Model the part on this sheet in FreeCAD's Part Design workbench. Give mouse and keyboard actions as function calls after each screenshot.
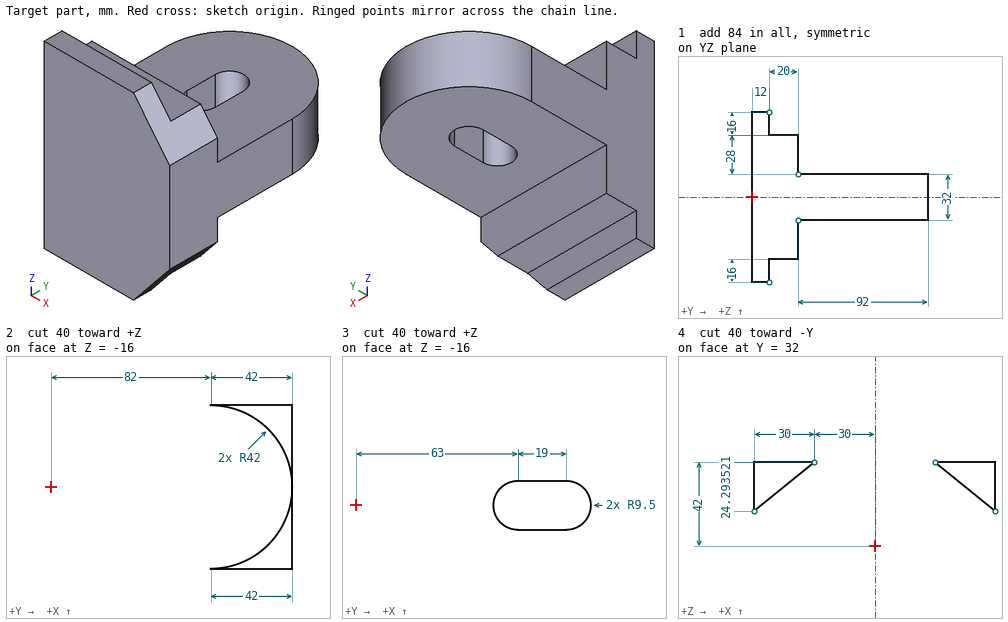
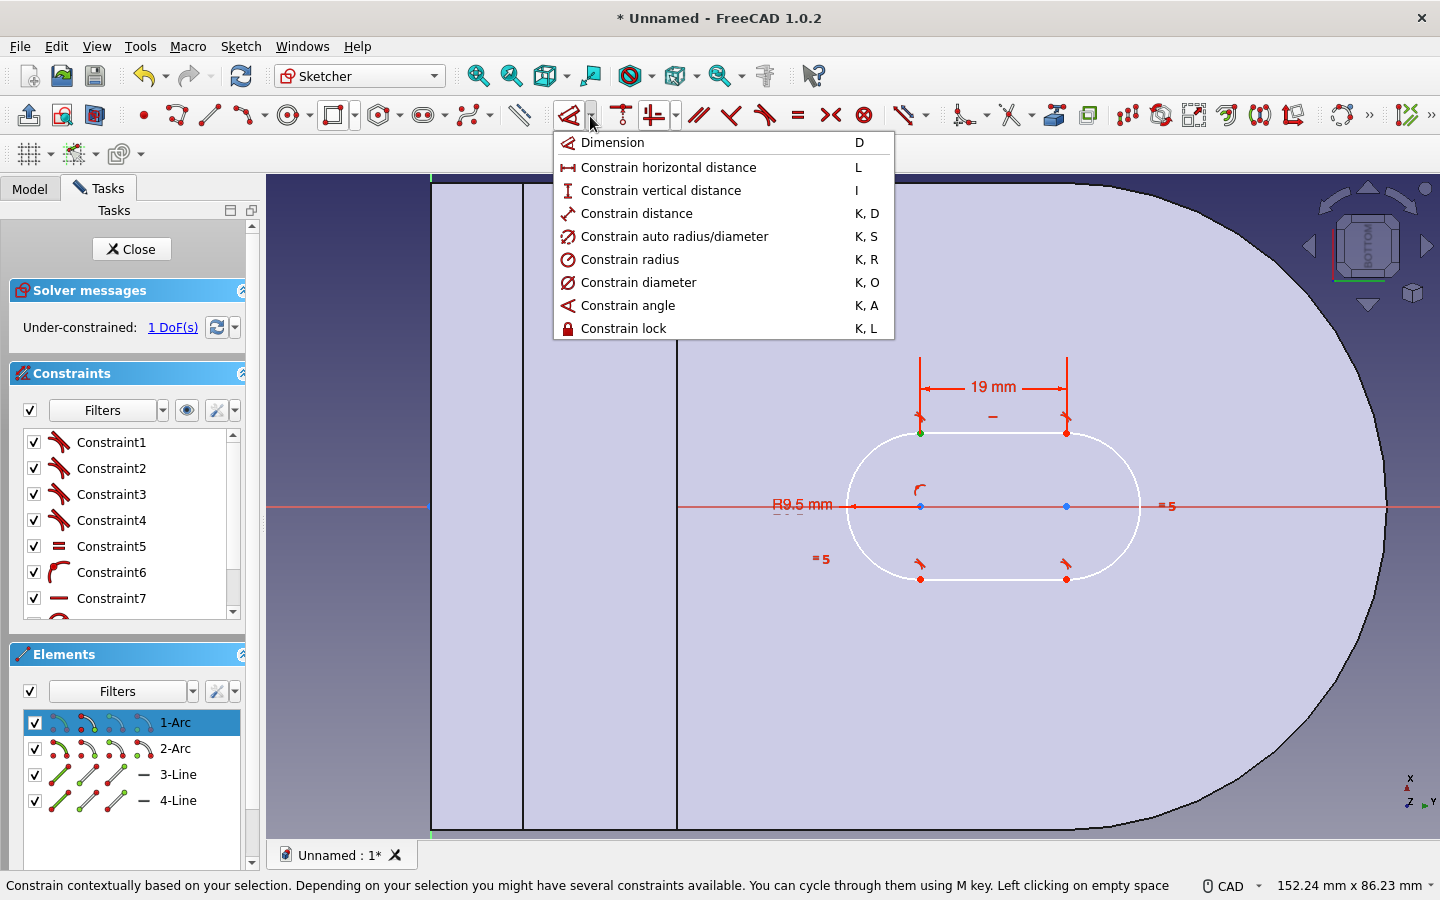
click(724, 168)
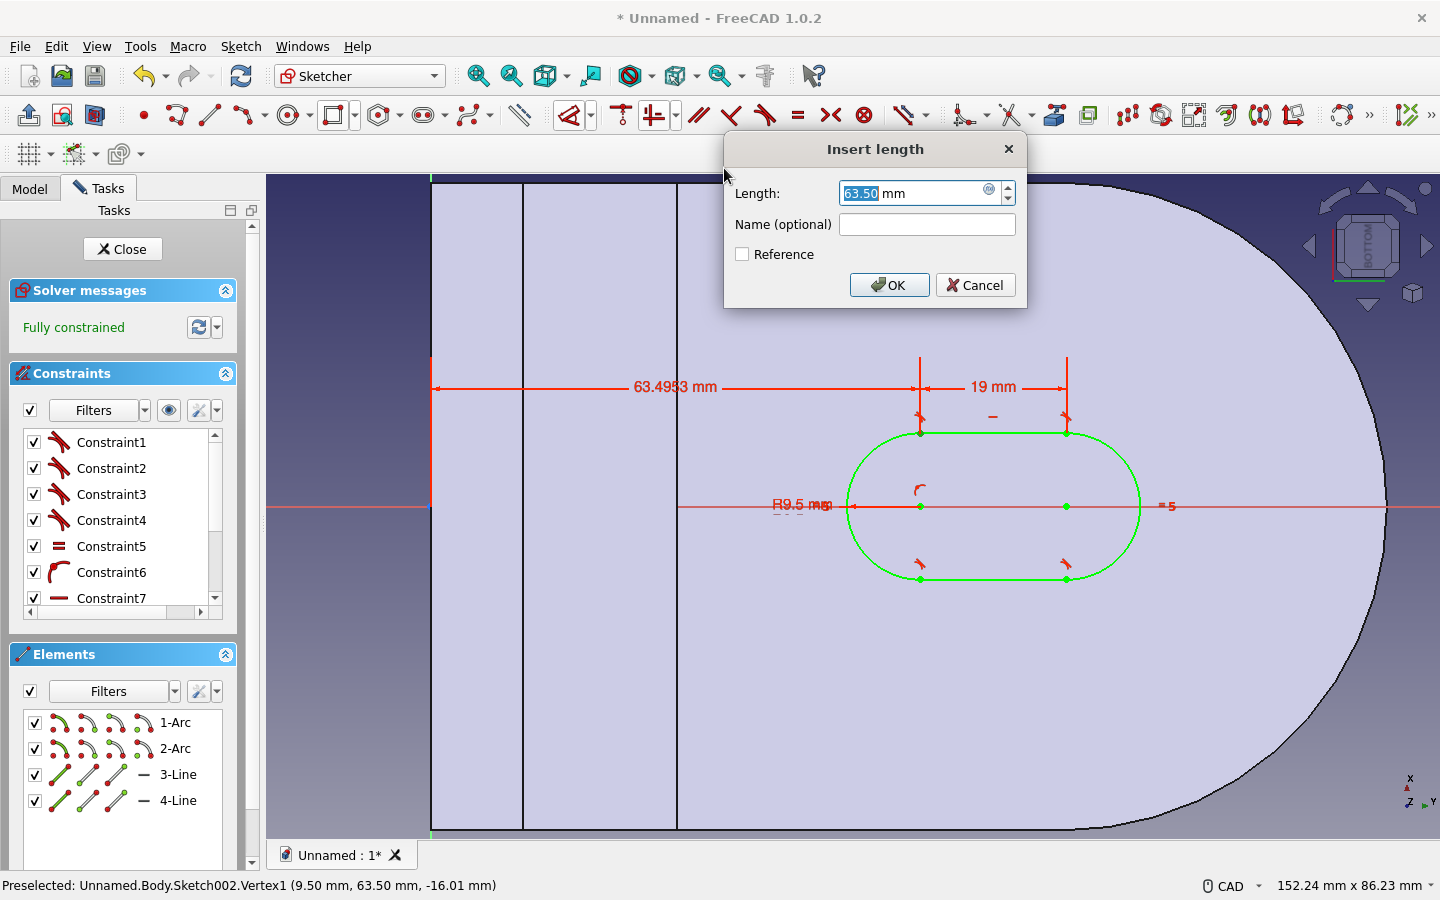
text(63)
key(Return)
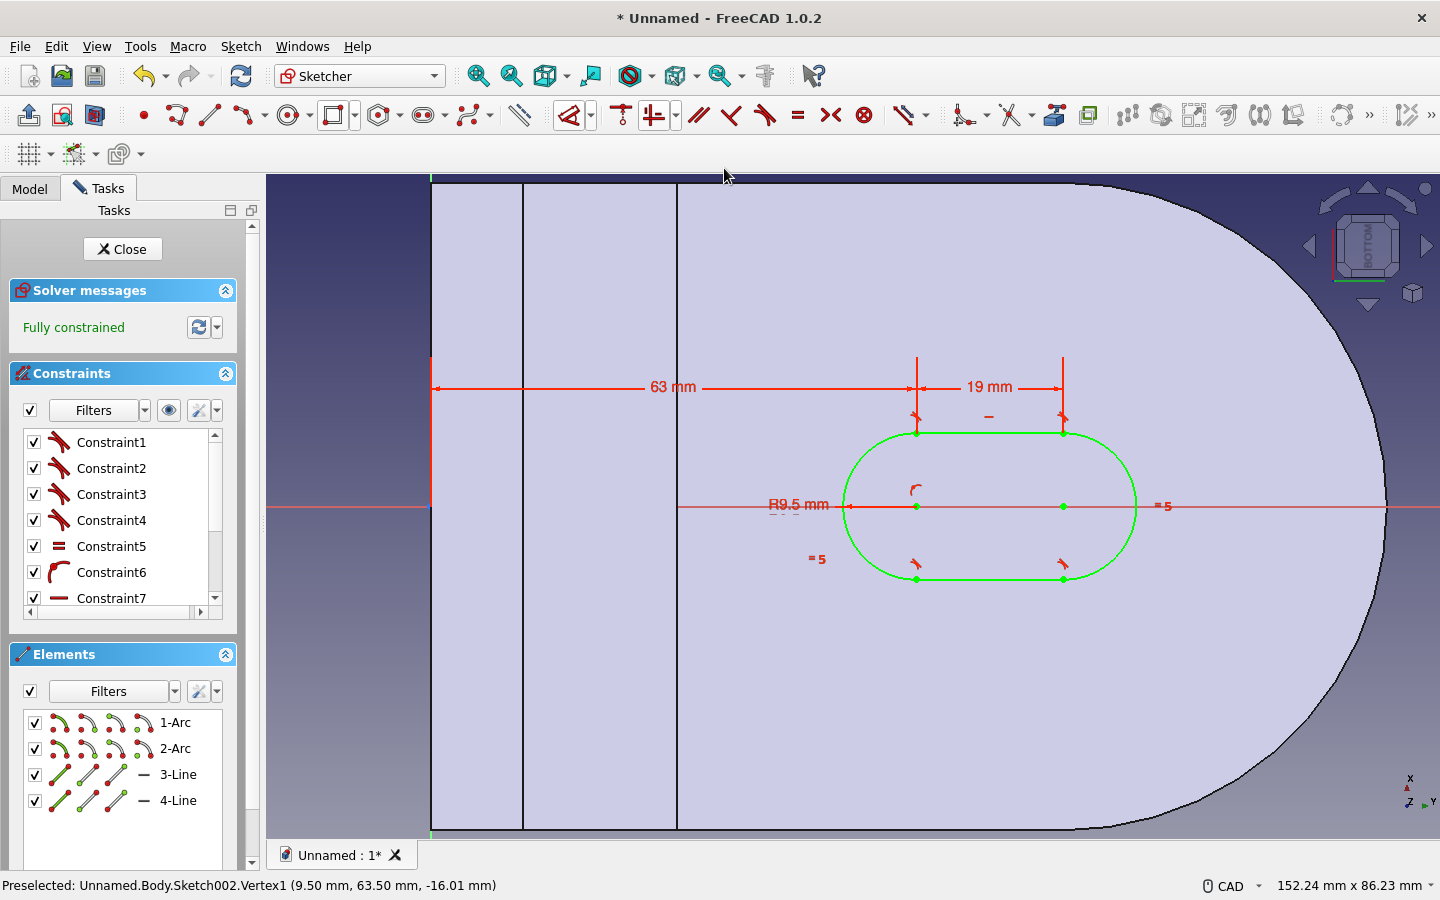
click(123, 249)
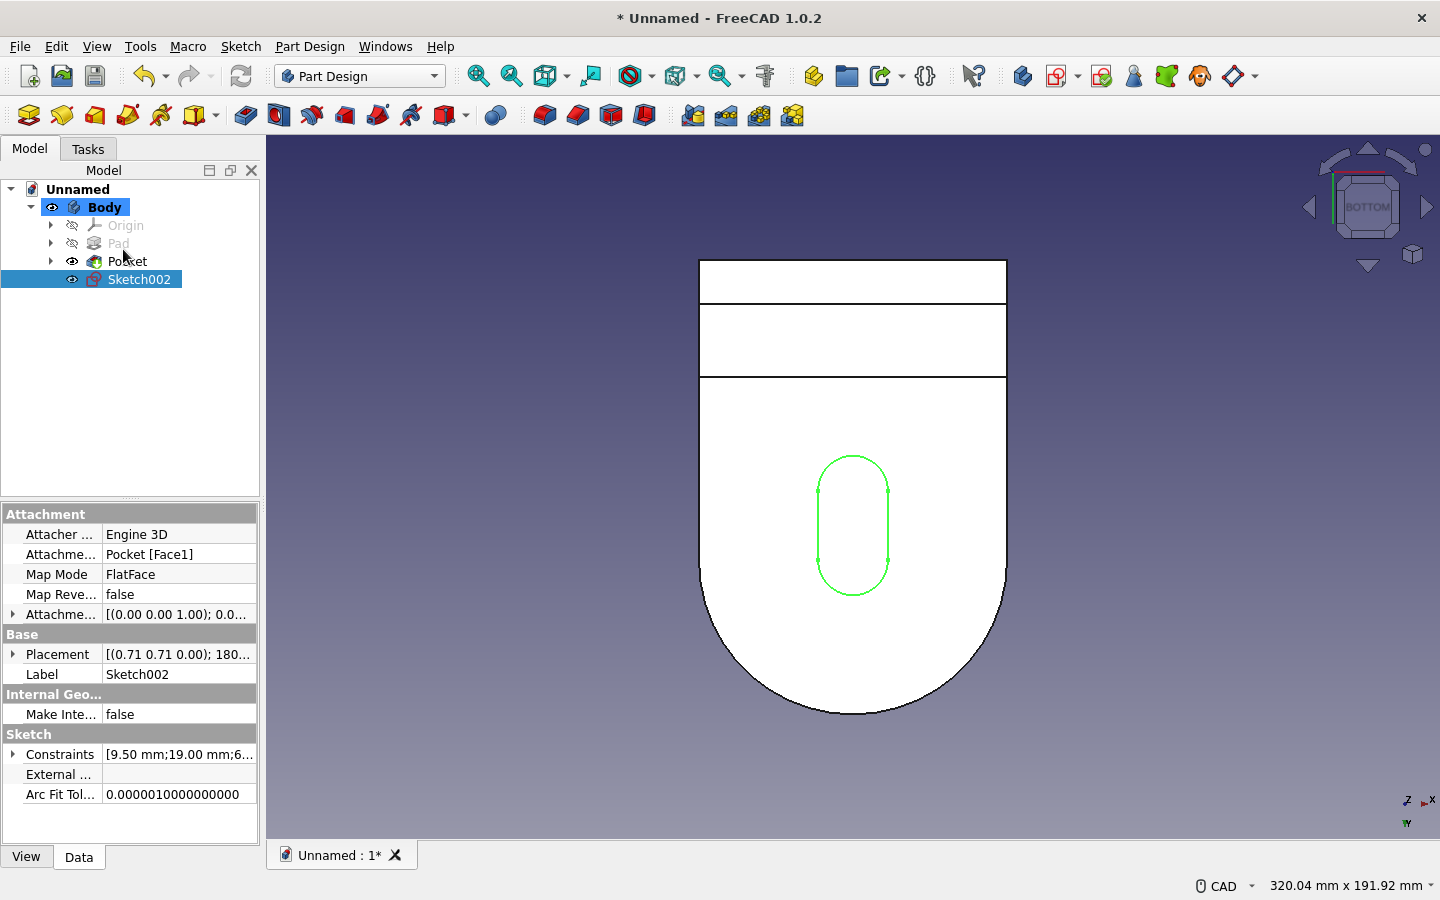
click(246, 116)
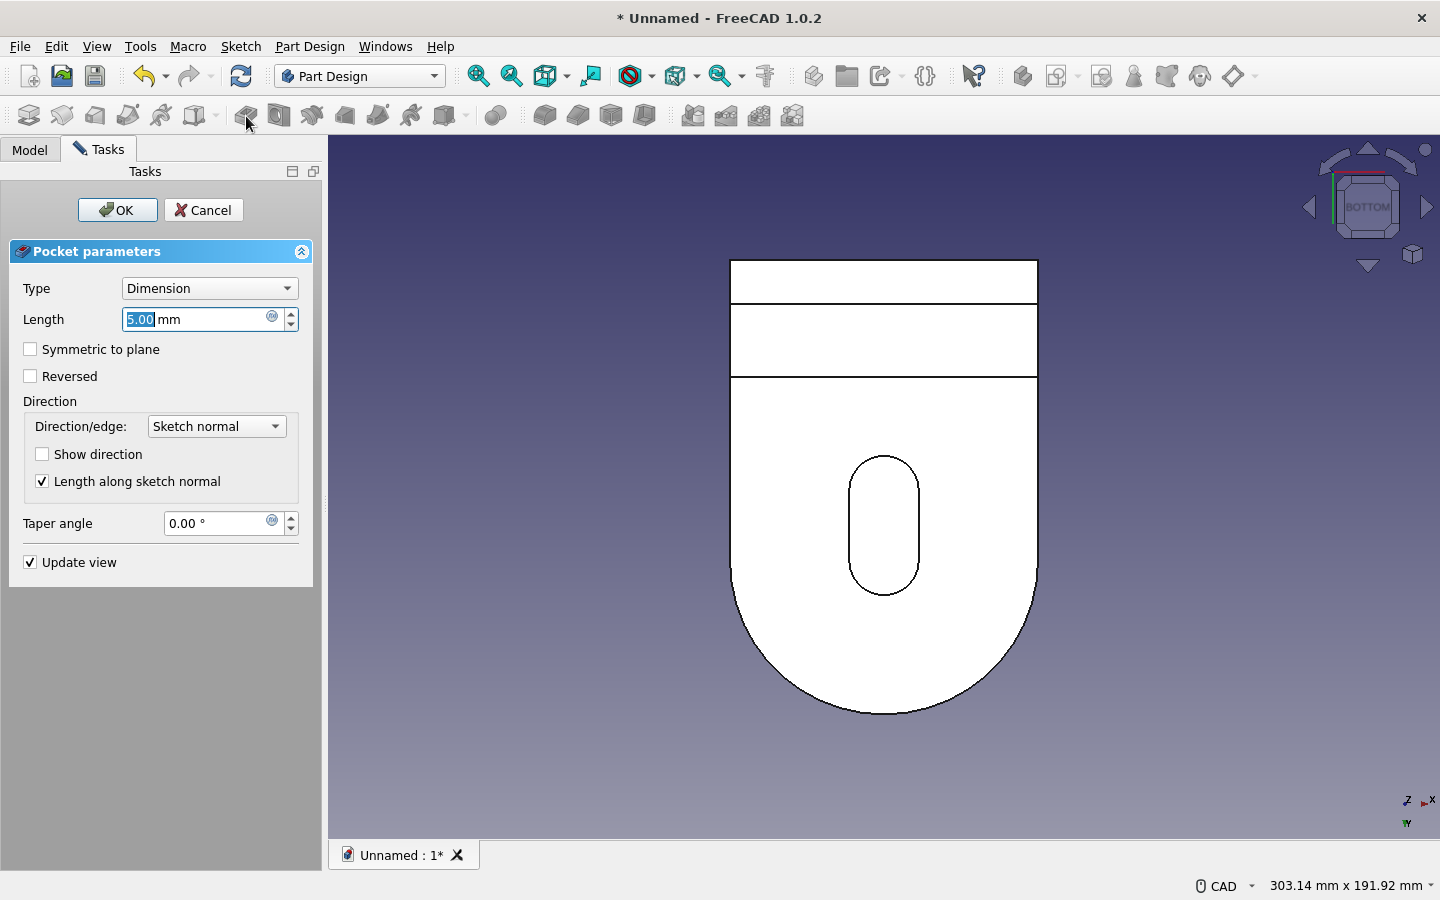
text(40)
key(Tab)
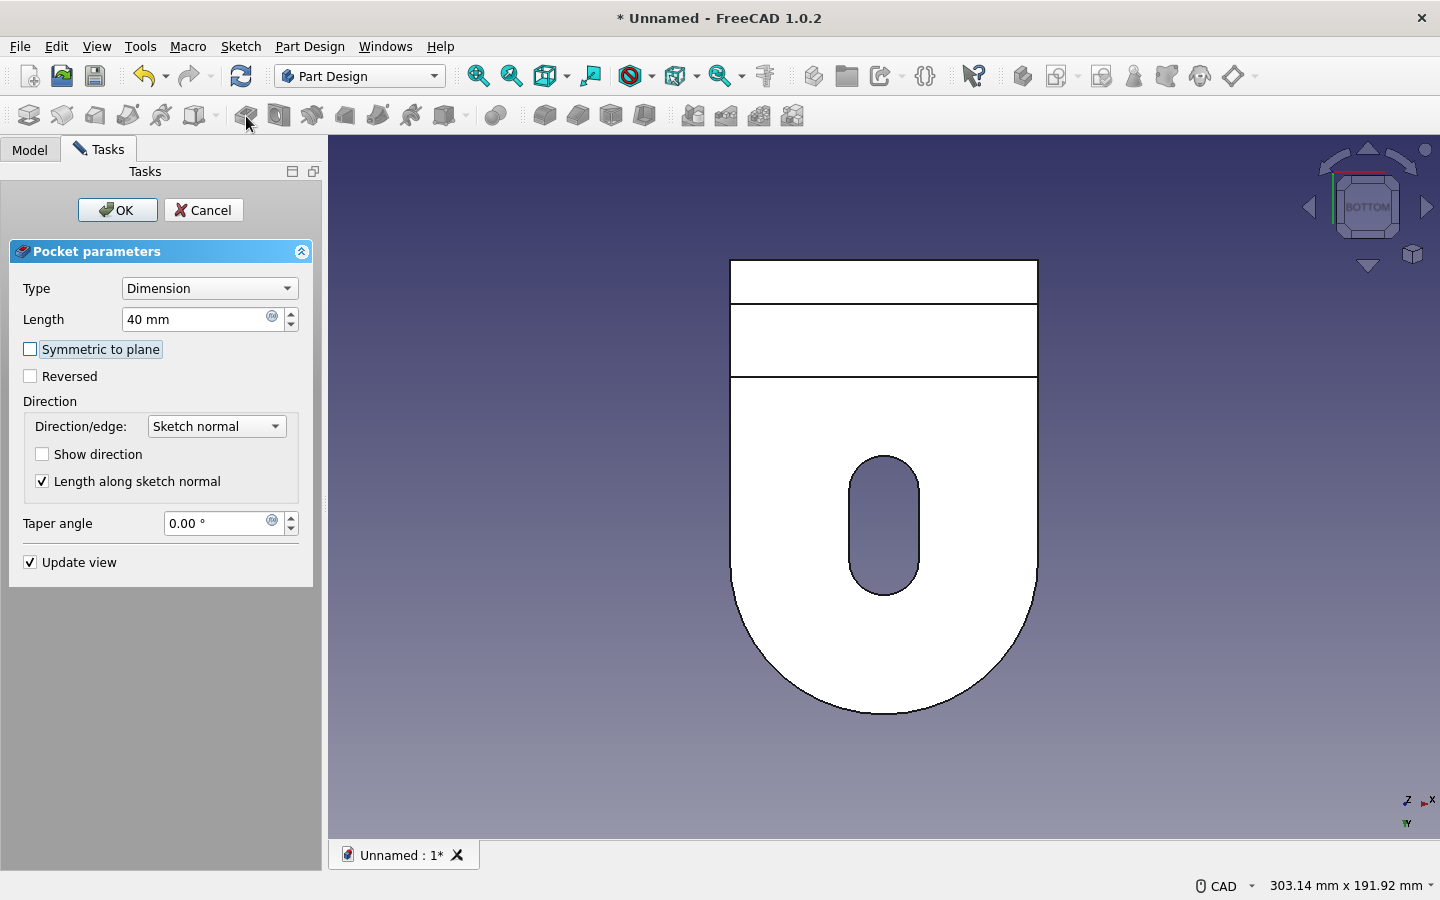
click(118, 210)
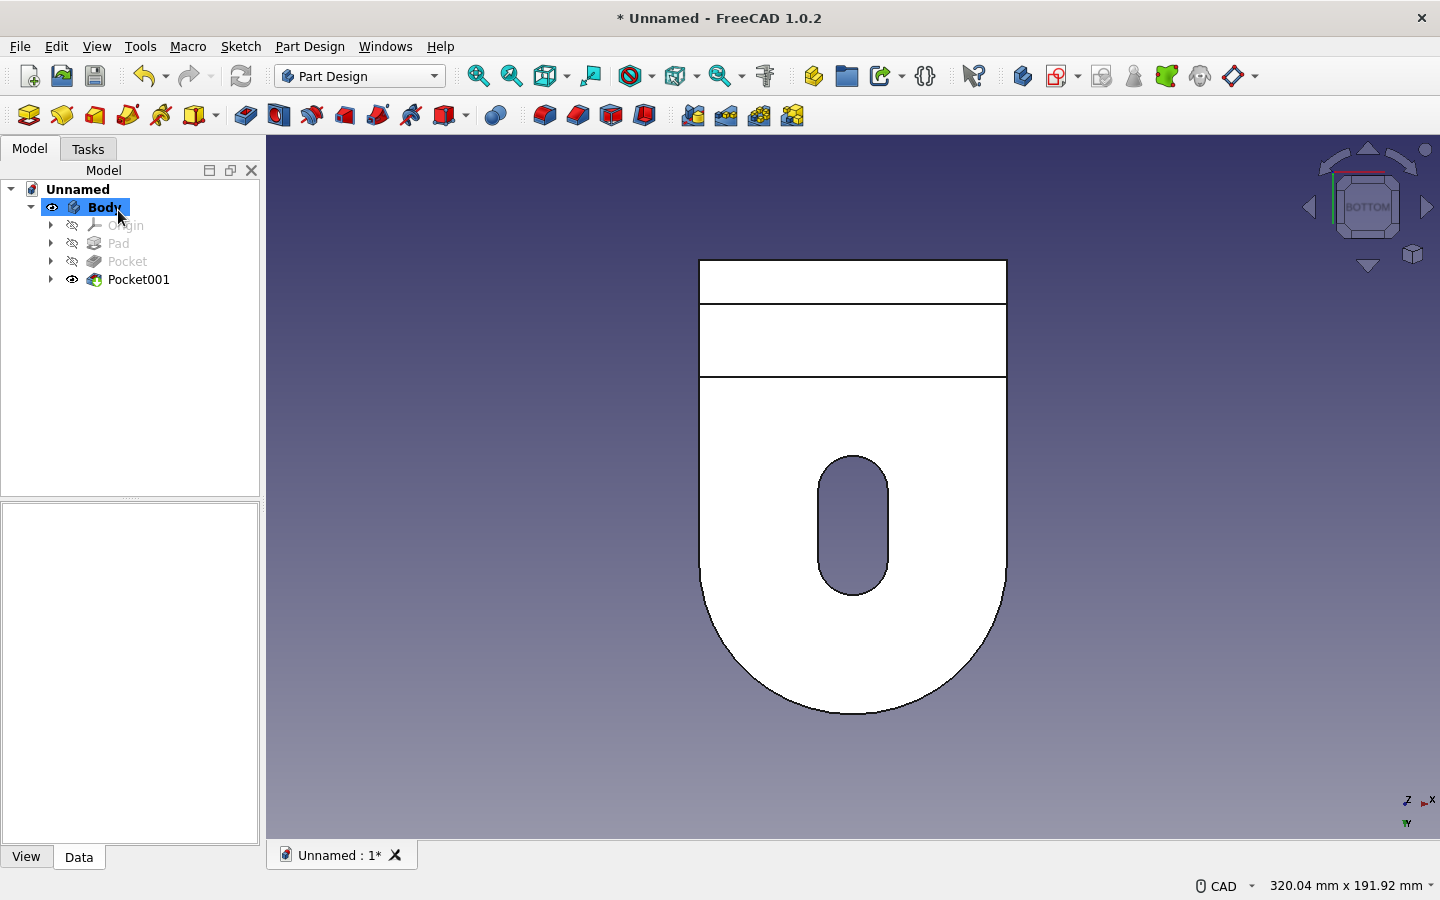
key(4)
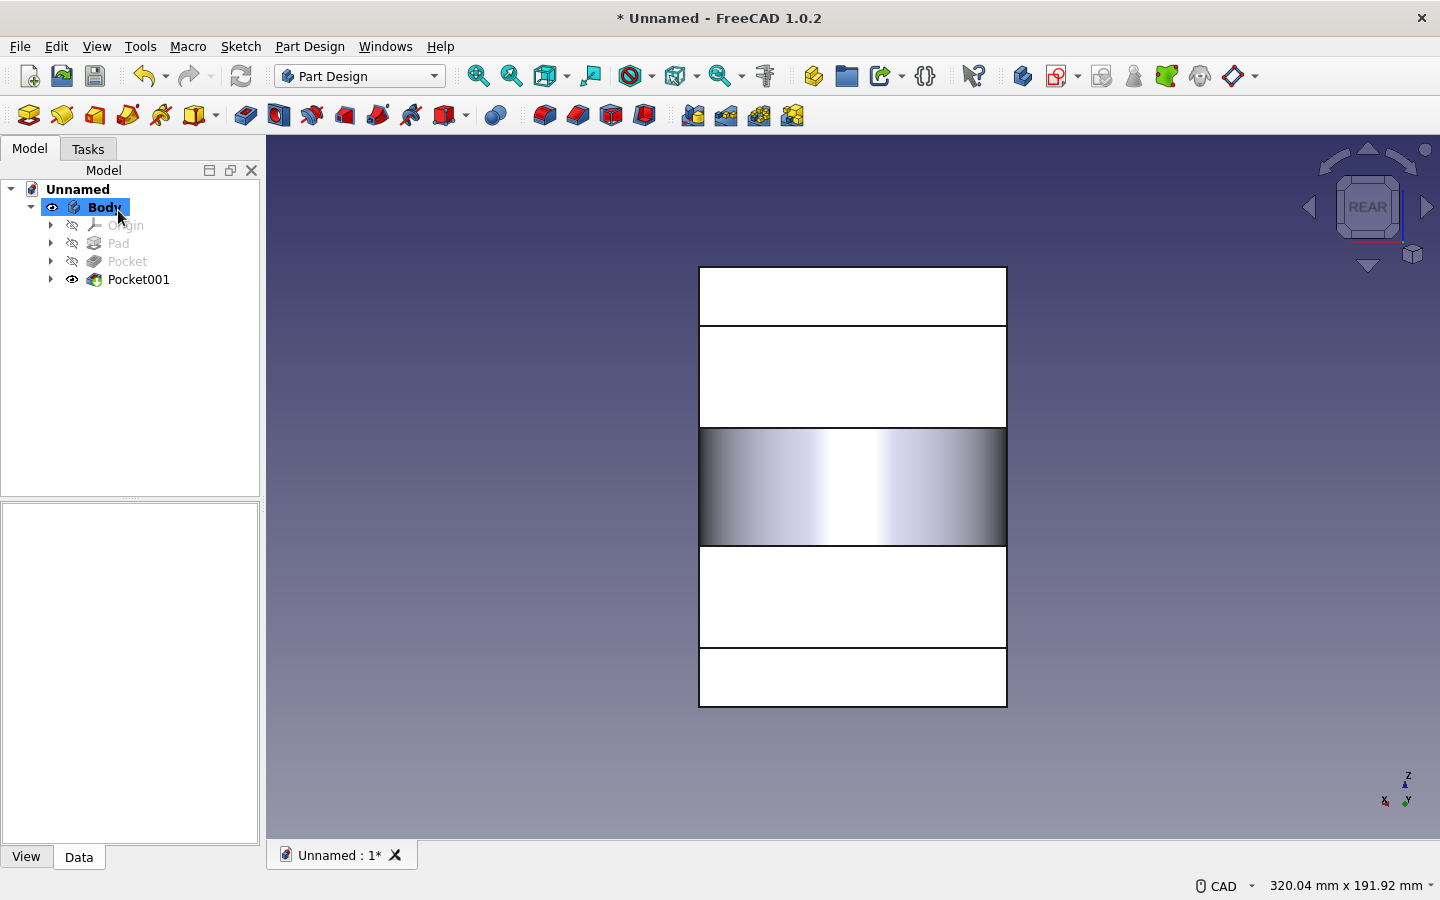
click(853, 596)